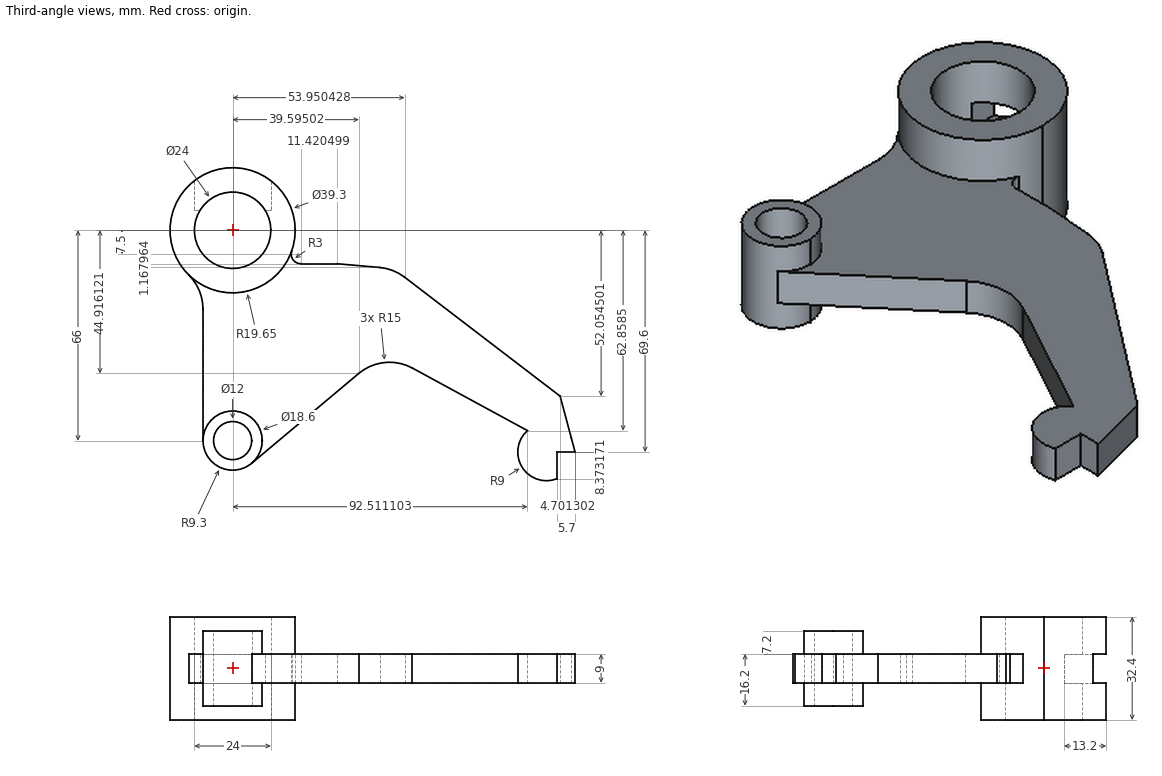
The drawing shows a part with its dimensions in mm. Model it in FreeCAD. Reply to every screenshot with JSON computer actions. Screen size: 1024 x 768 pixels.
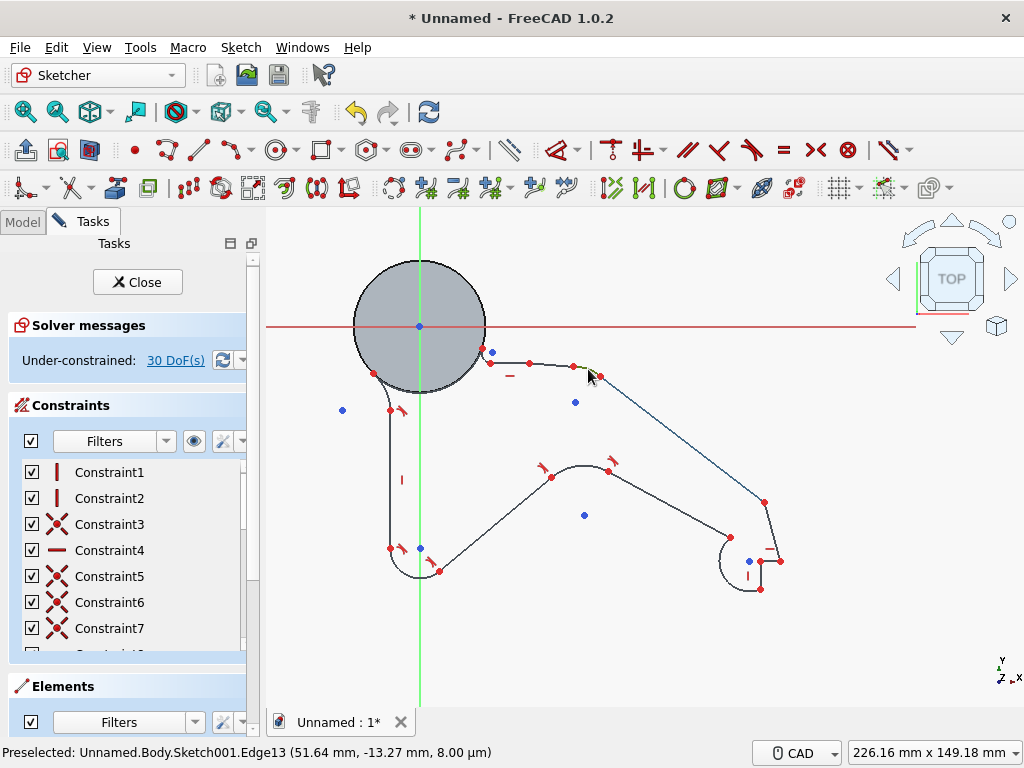
{"action": "key", "text": "t"}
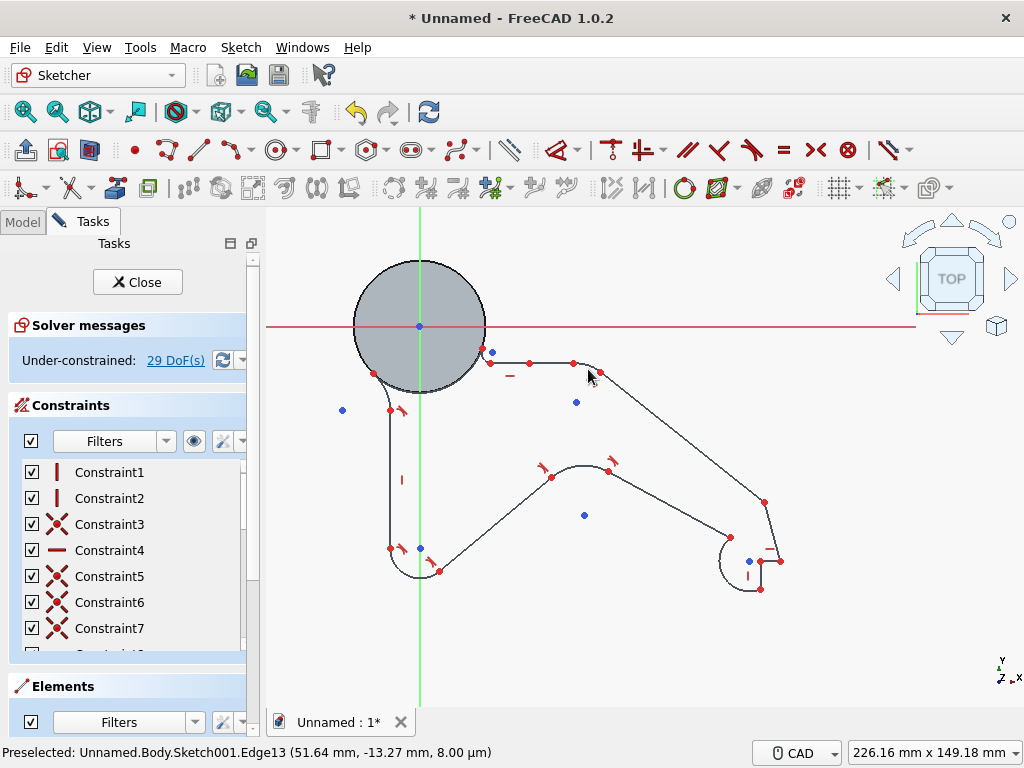
{"action": "left_click", "coordinate": [561, 363]}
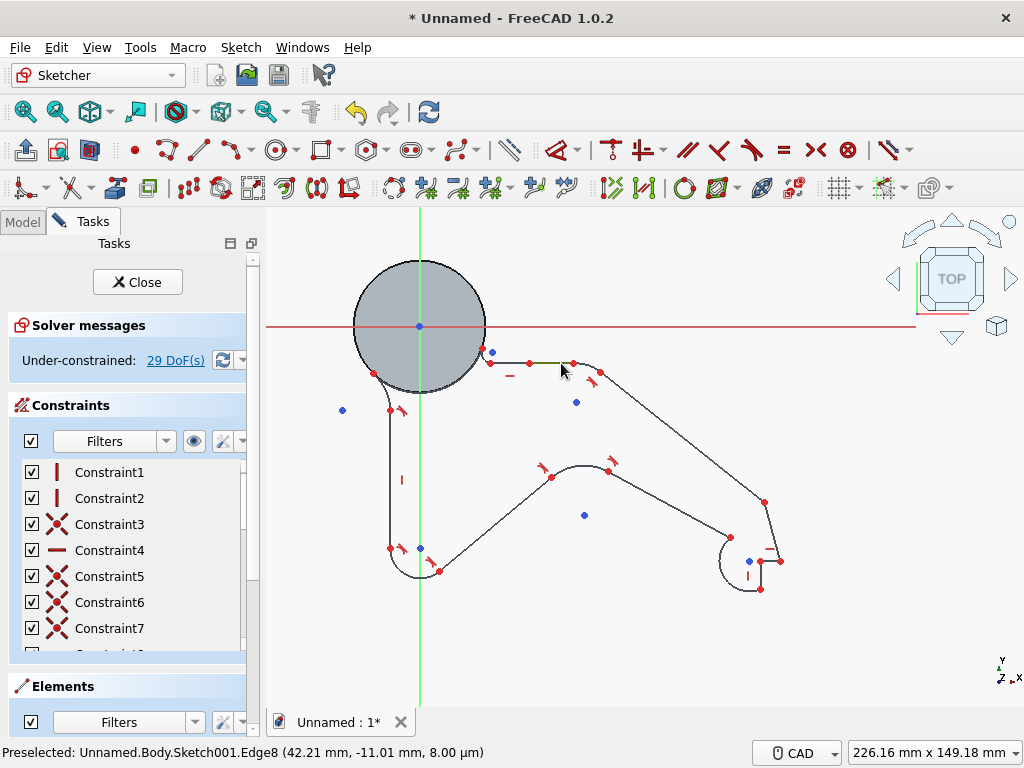
{"action": "left_click", "coordinate": [588, 365]}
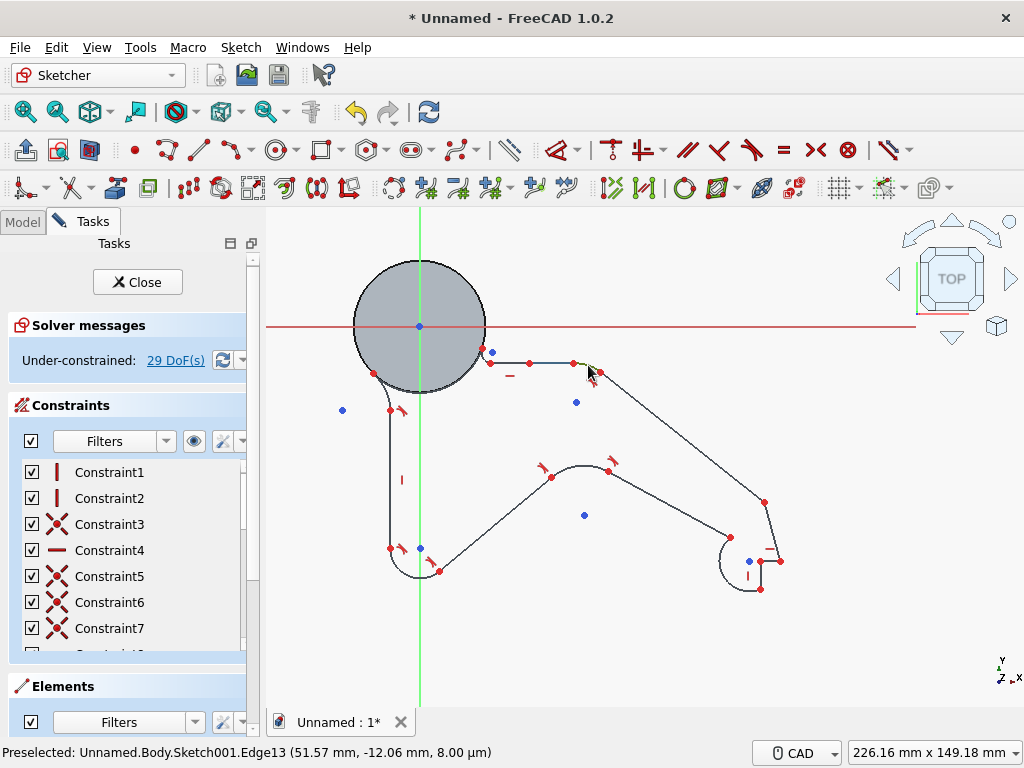
{"action": "key", "text": "t"}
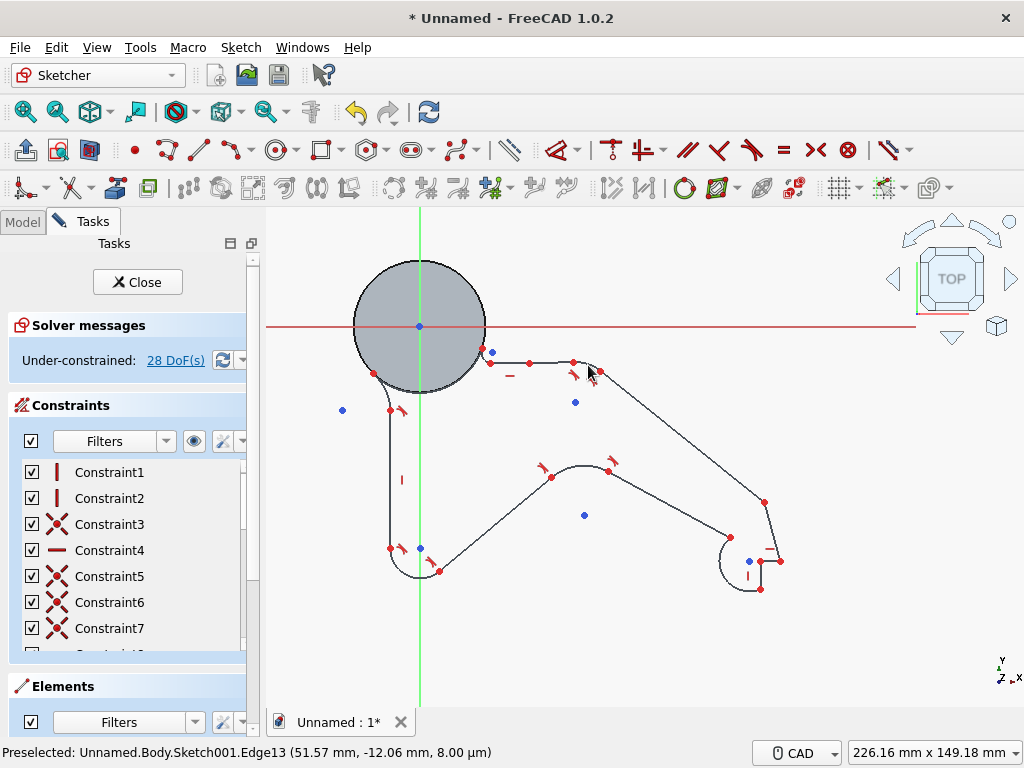
{"action": "left_click", "coordinate": [518, 363]}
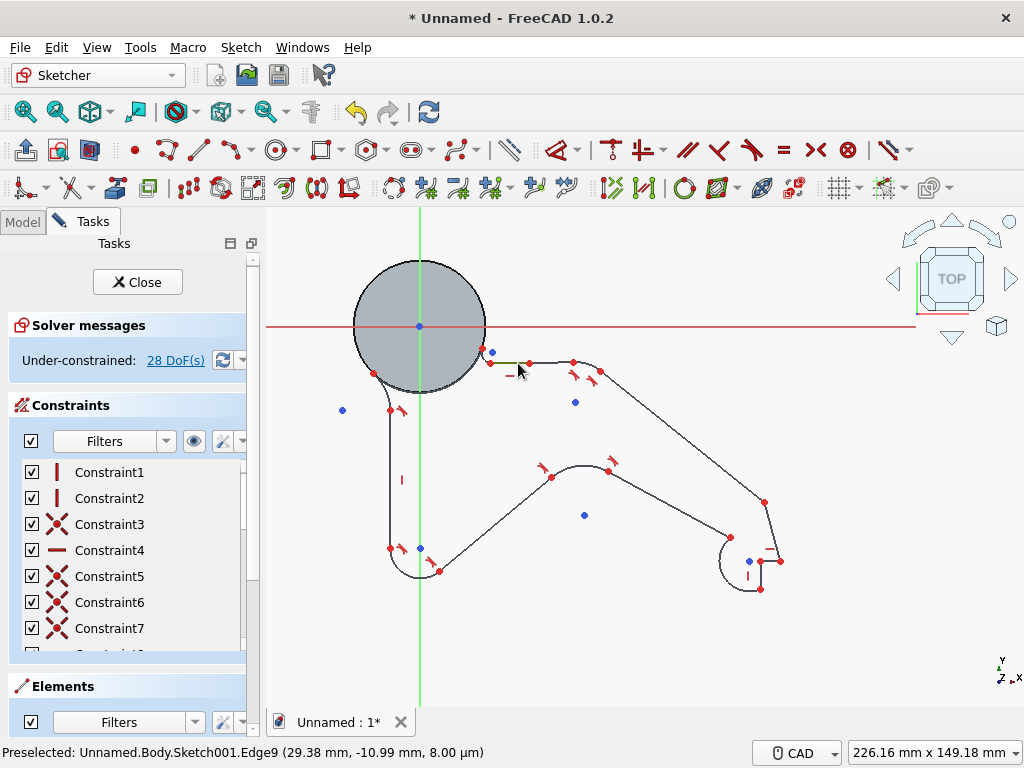
{"action": "scroll", "coordinate": [486, 361], "scroll_direction": "up", "scroll_amount": 5}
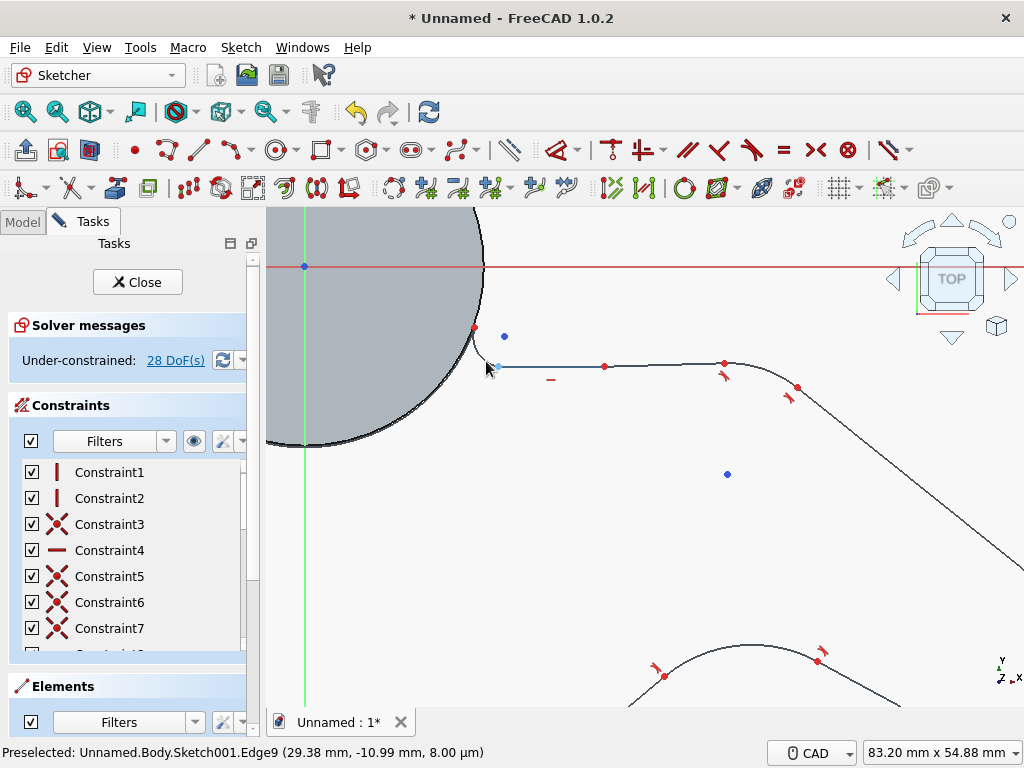
{"action": "left_click", "coordinate": [485, 360]}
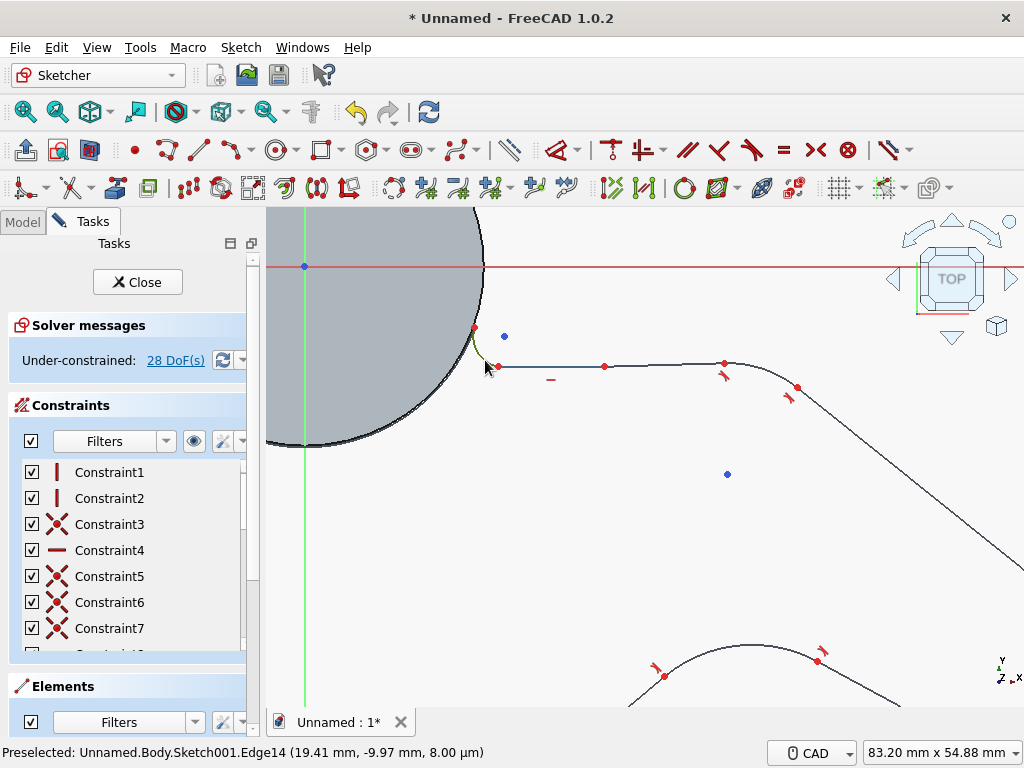
{"action": "left_click", "coordinate": [752, 150]}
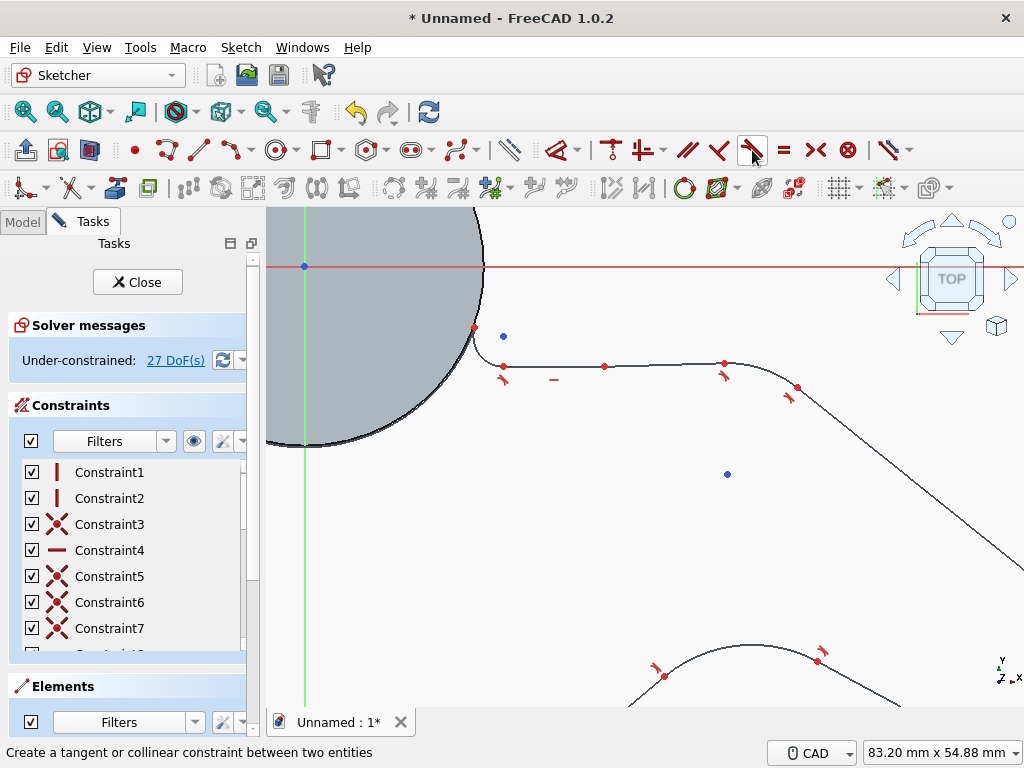
{"action": "left_click", "coordinate": [488, 362]}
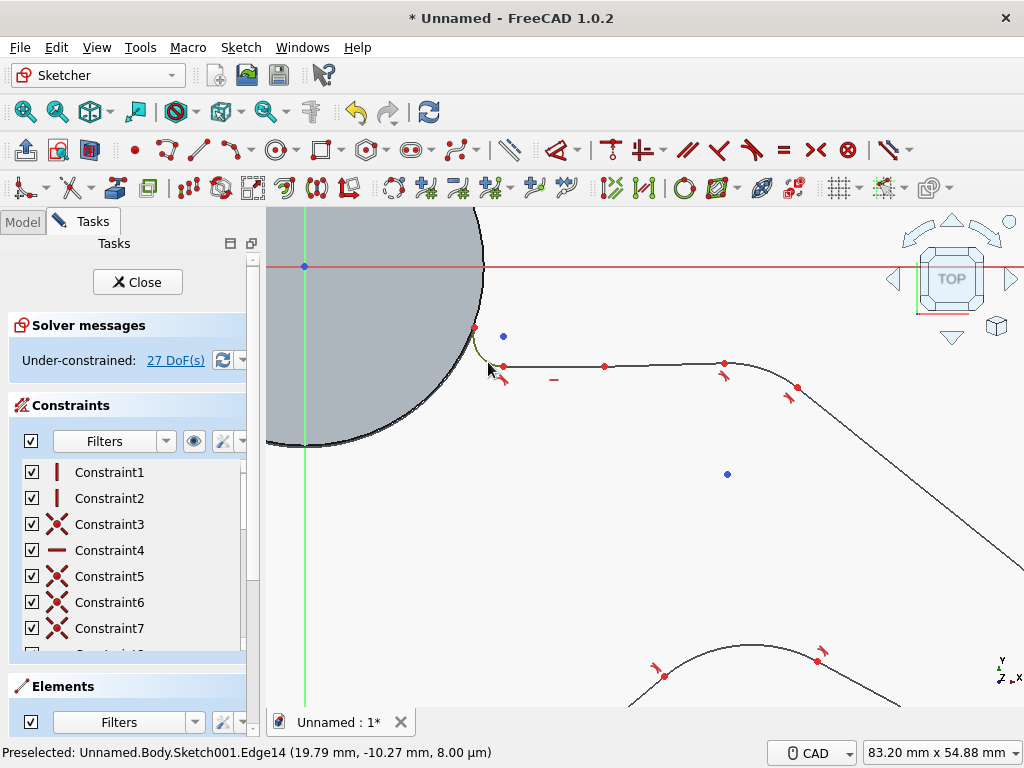
{"action": "left_click", "coordinate": [410, 413]}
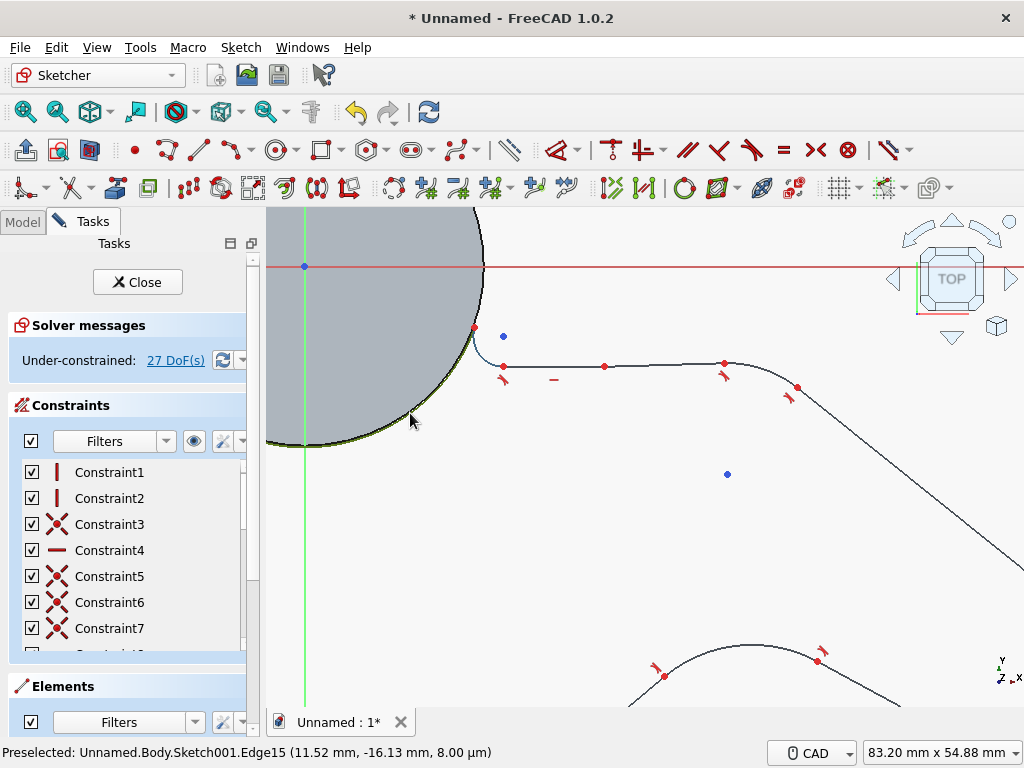
{"action": "left_click", "coordinate": [752, 150]}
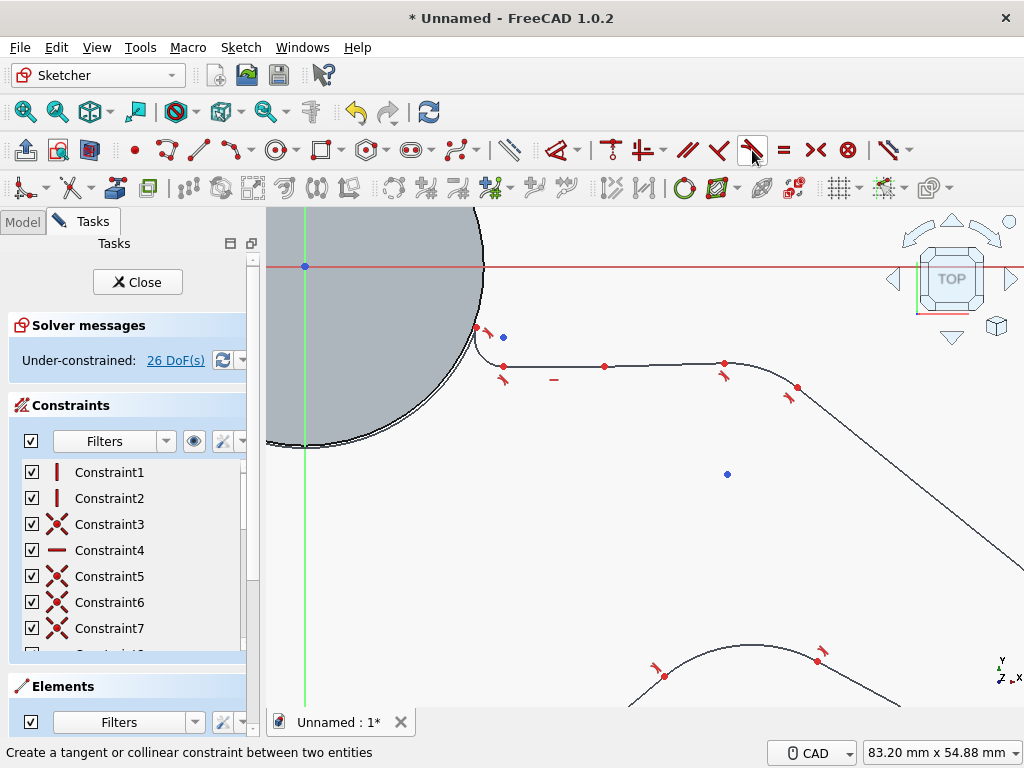
{"action": "left_click", "coordinate": [412, 414]}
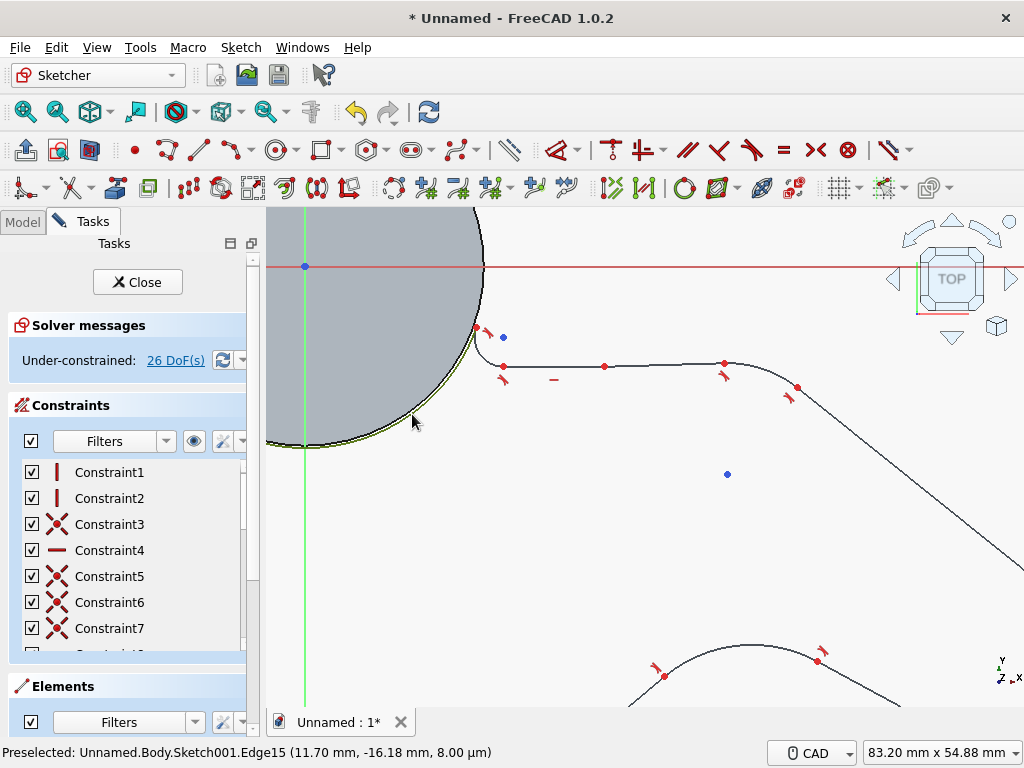
{"action": "scroll", "coordinate": [486, 361], "scroll_direction": "down", "scroll_amount": 5}